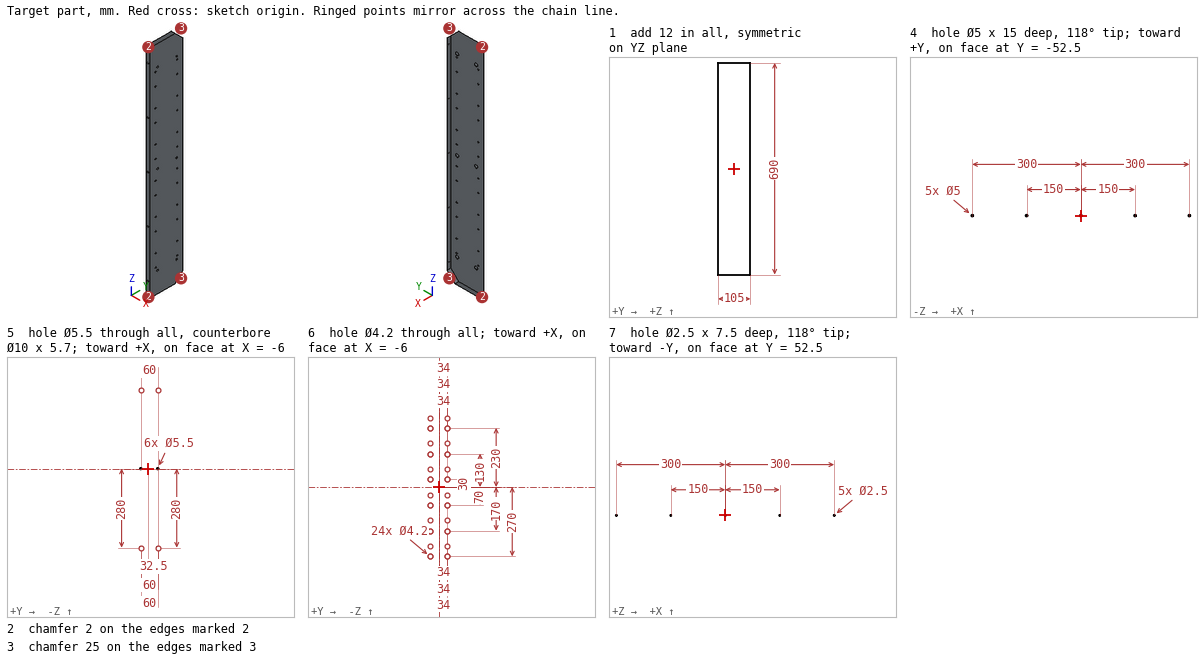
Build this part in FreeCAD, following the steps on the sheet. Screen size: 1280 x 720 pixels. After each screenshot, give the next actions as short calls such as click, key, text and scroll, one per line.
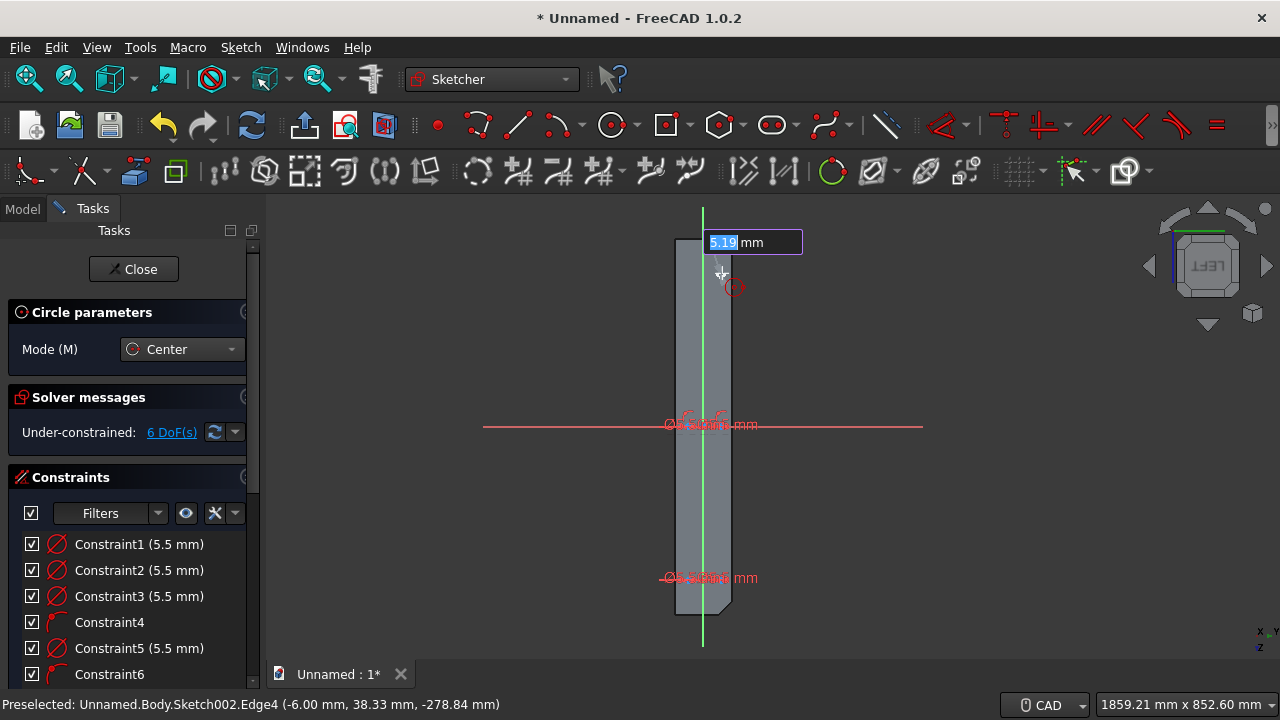
text(5.5)
key(Return)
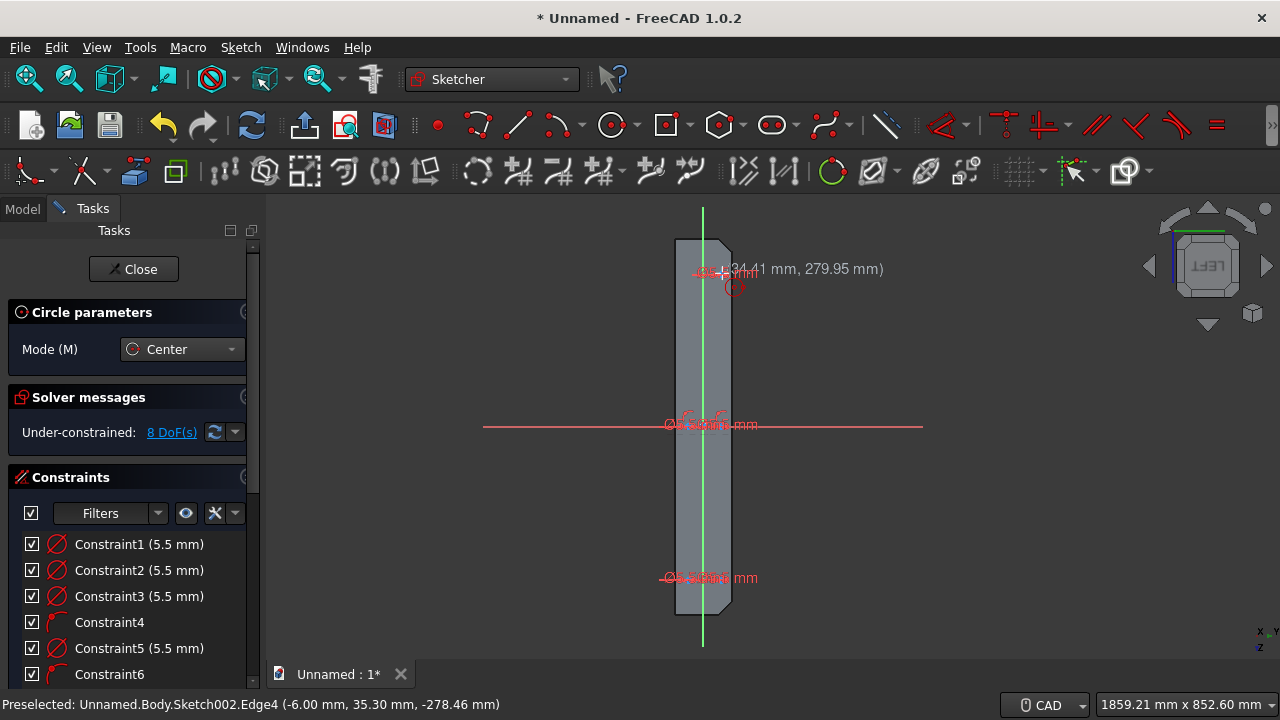
scroll(688, 274, up, 14)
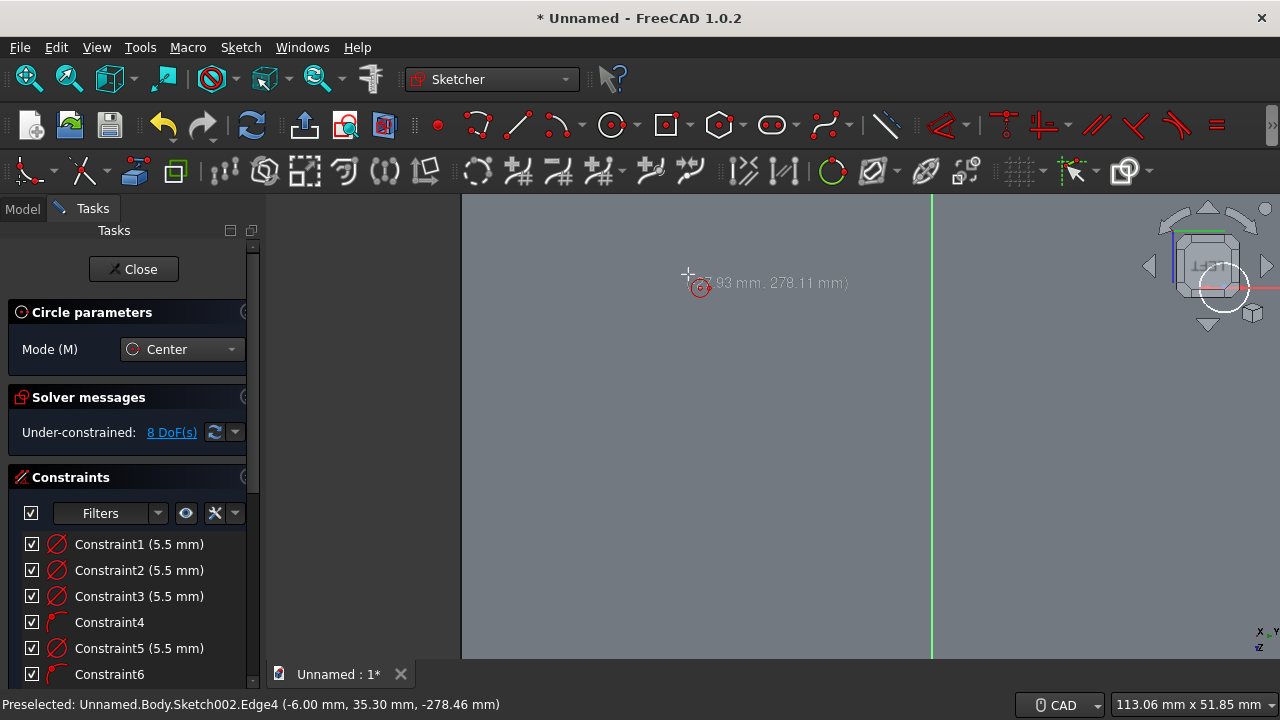
scroll(688, 274, down, 14)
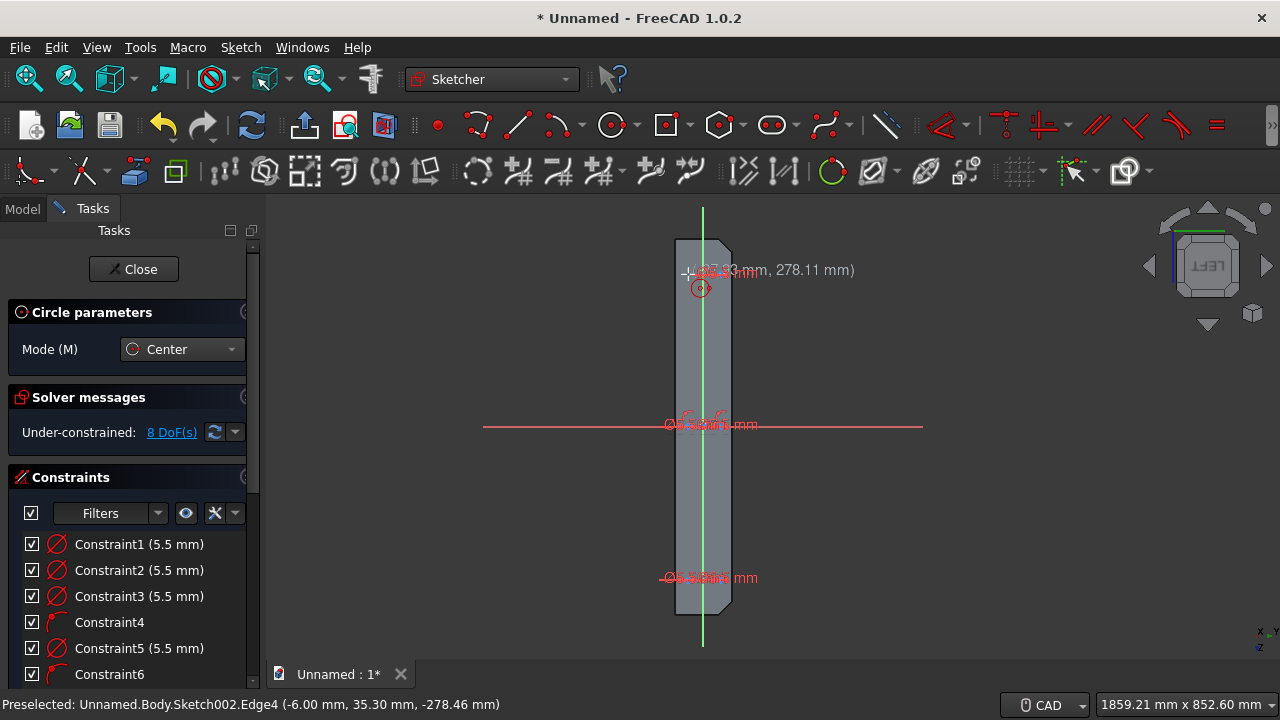
click(688, 274)
move(687, 273)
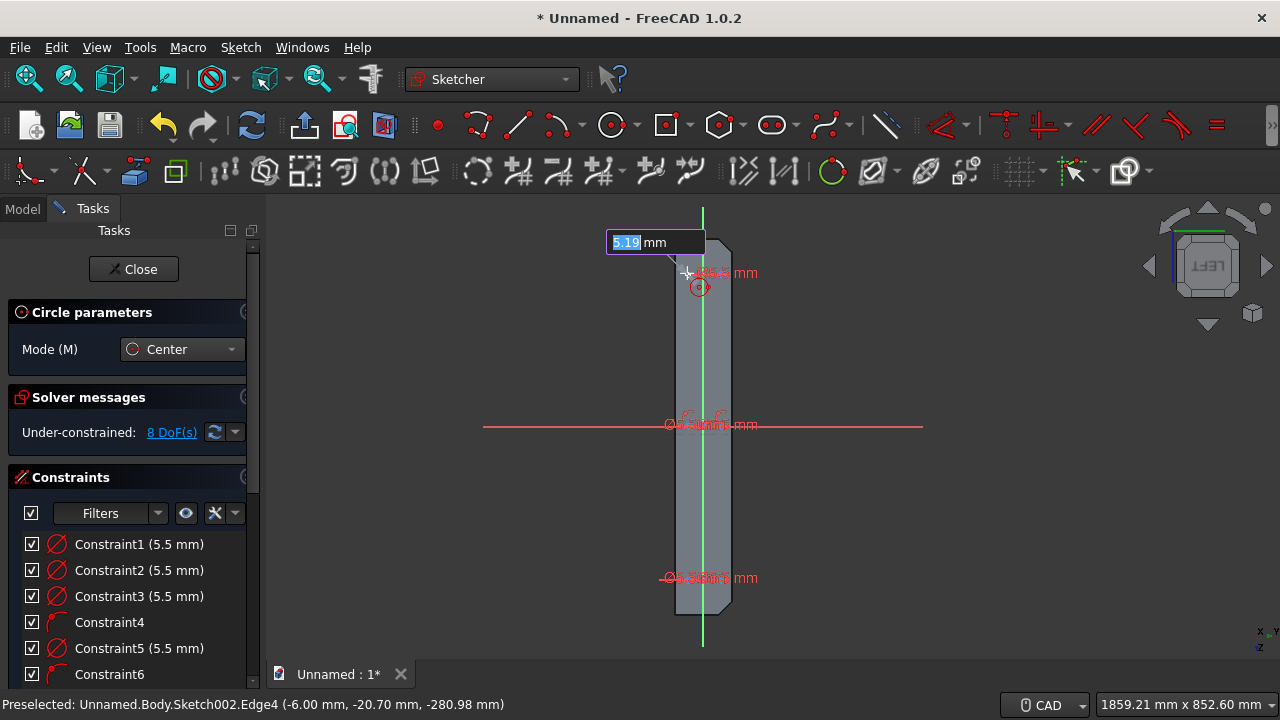
text(5.5)
key(Return)
key(Escape)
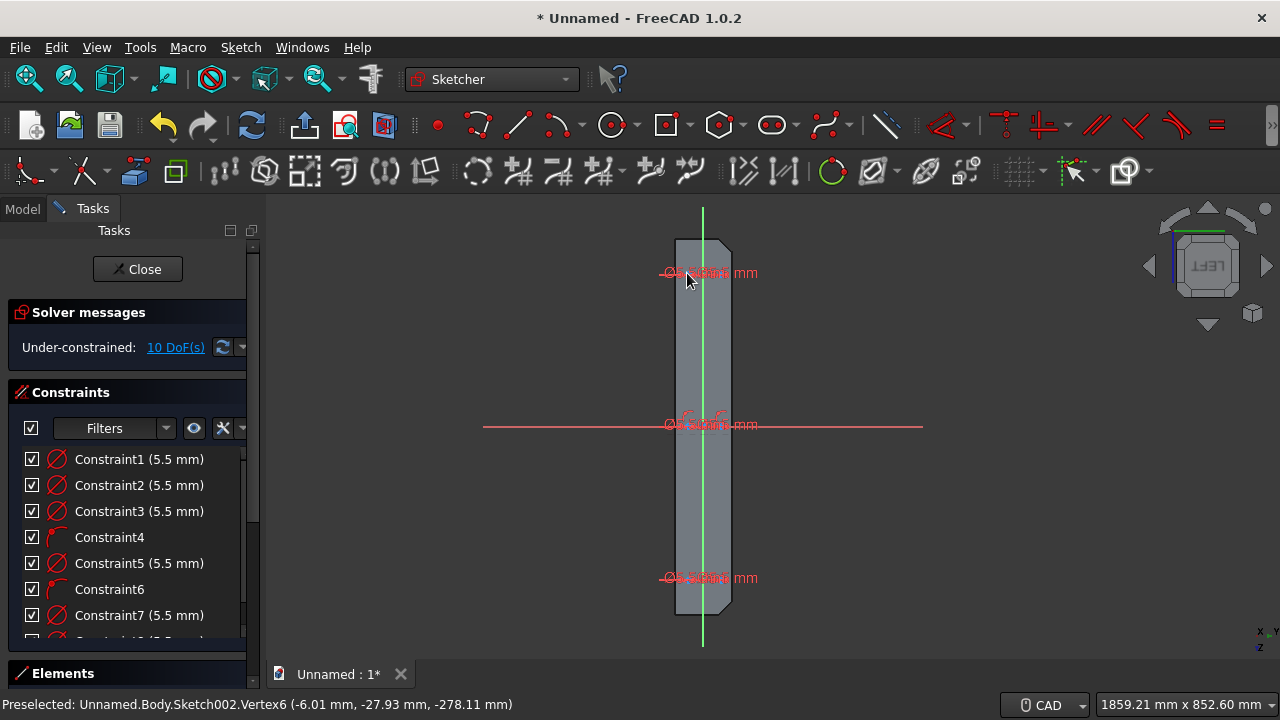
click(721, 580)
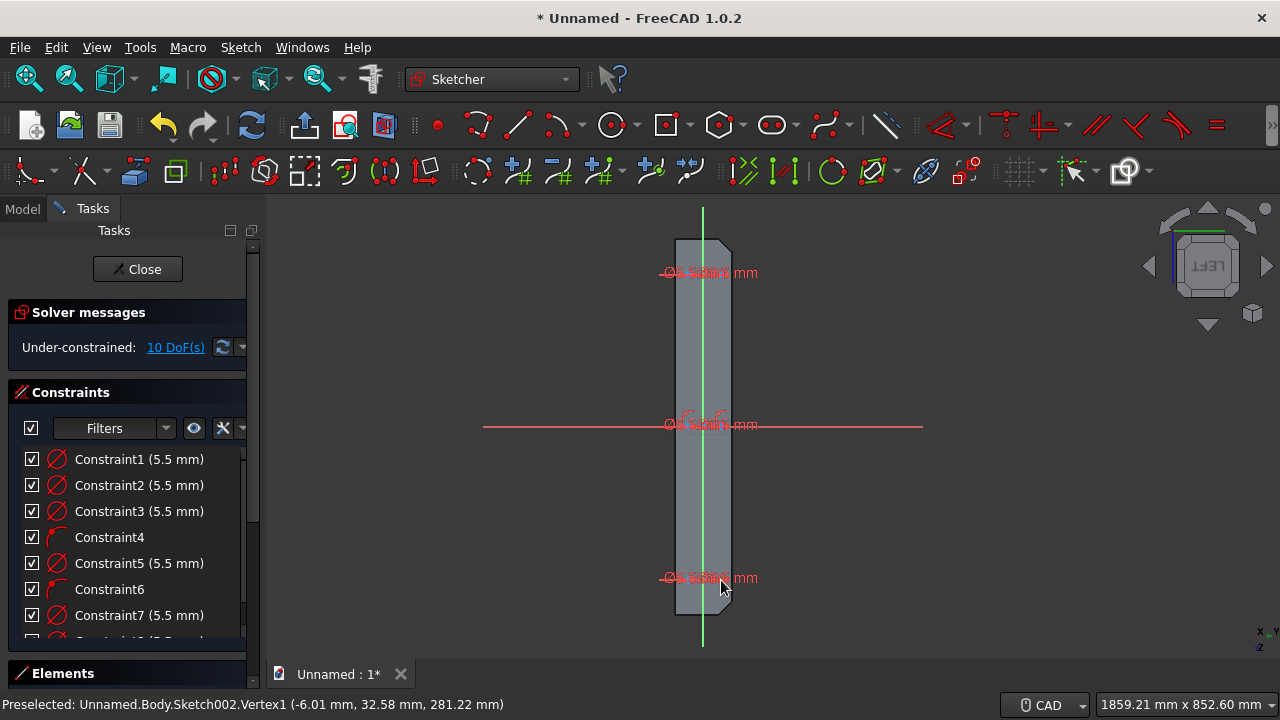
click(721, 275)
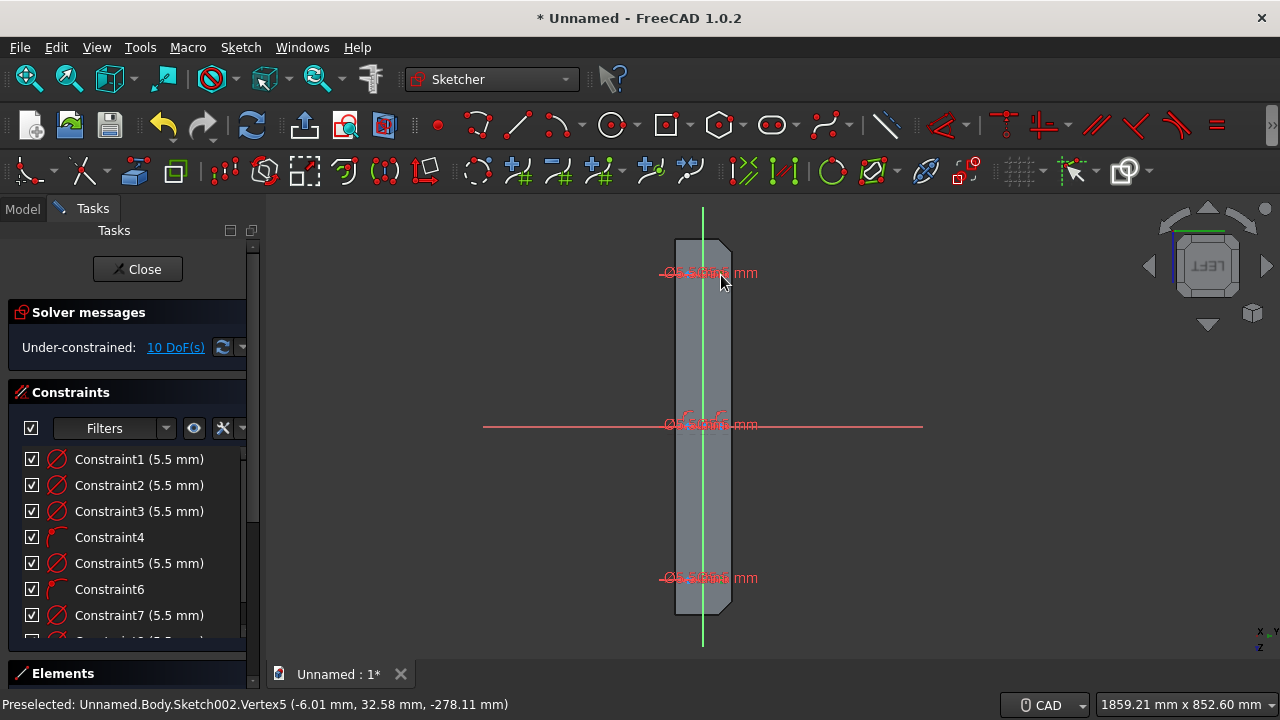
click(529, 427)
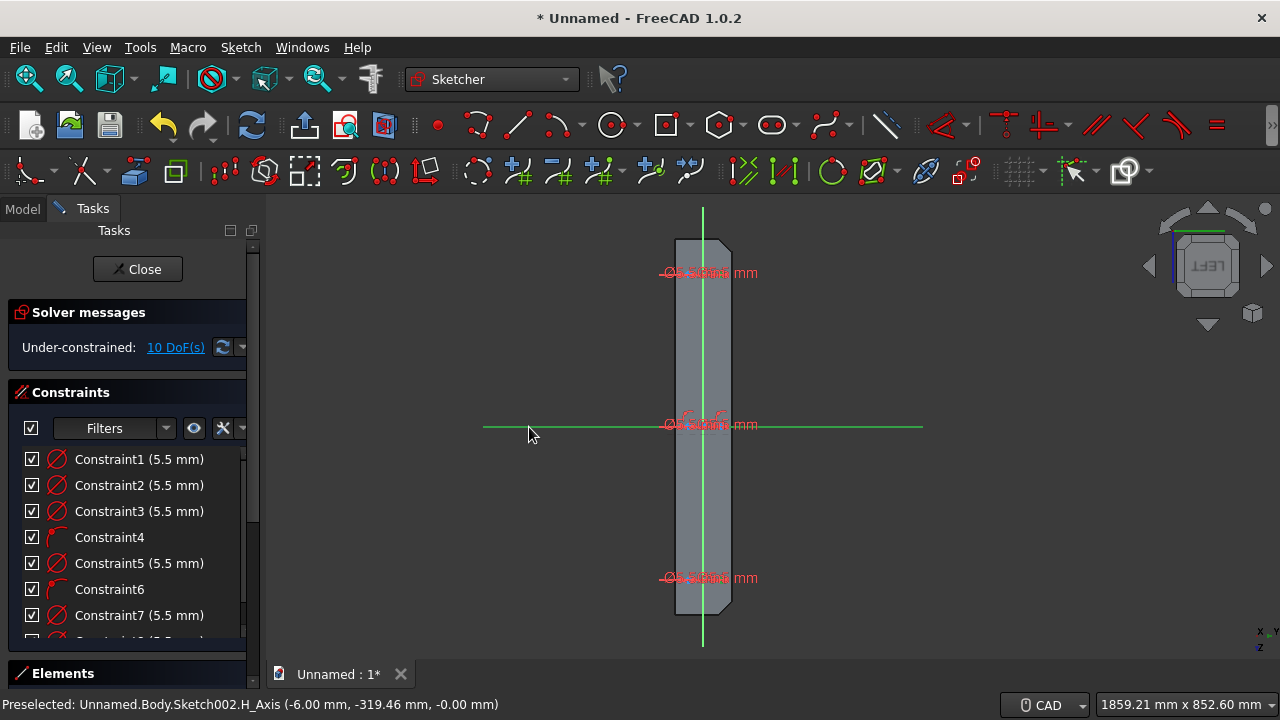
key(s)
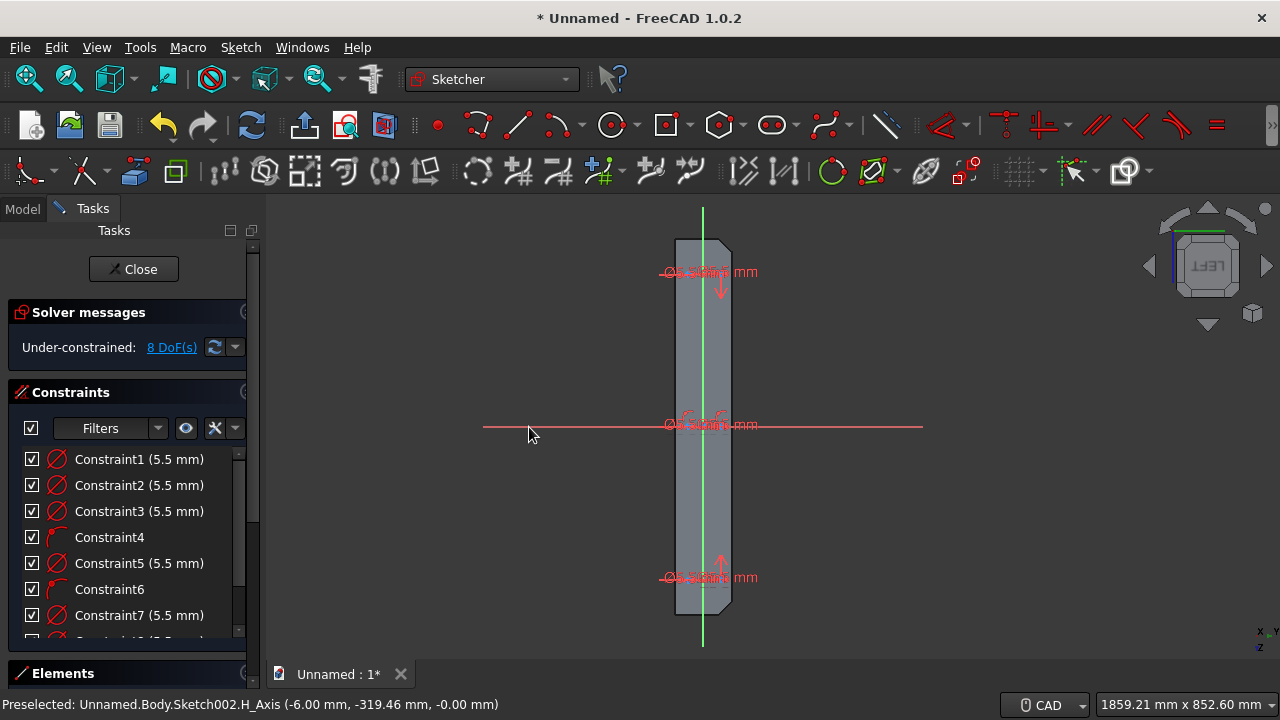
click(688, 580)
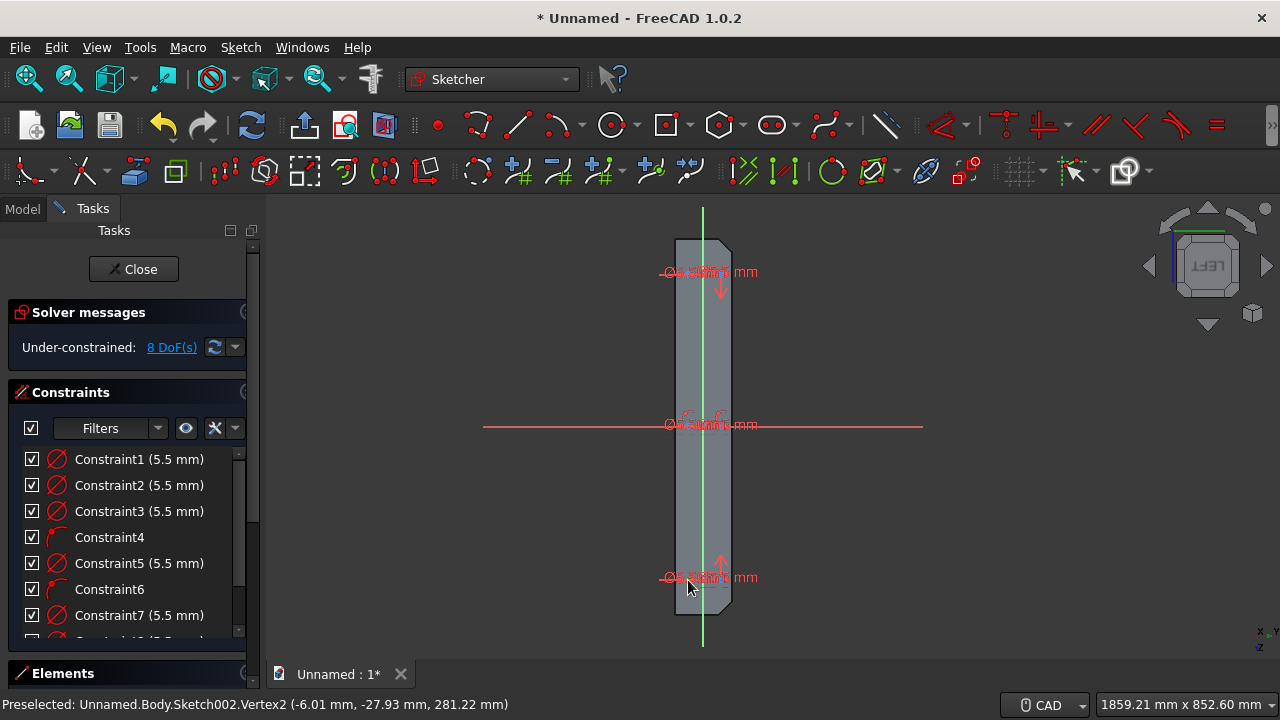
click(688, 275)